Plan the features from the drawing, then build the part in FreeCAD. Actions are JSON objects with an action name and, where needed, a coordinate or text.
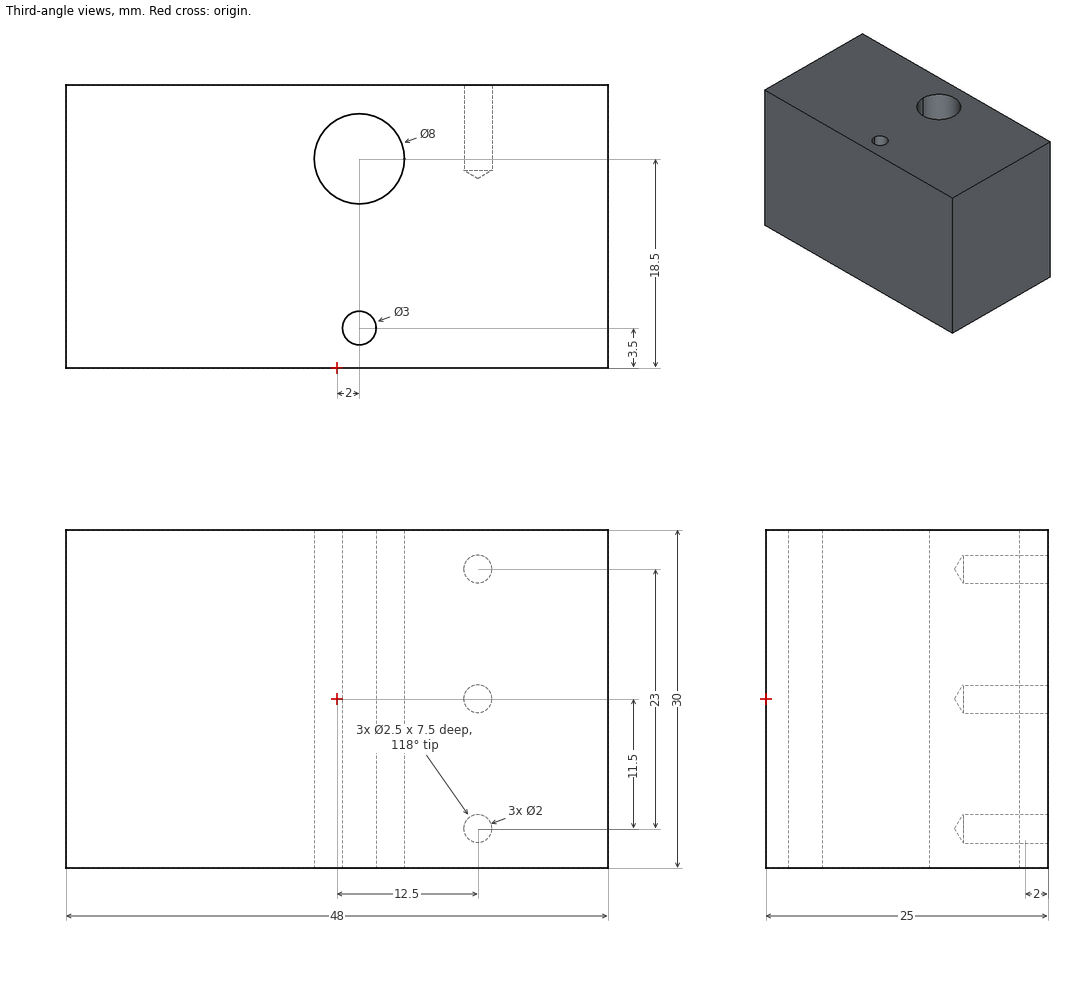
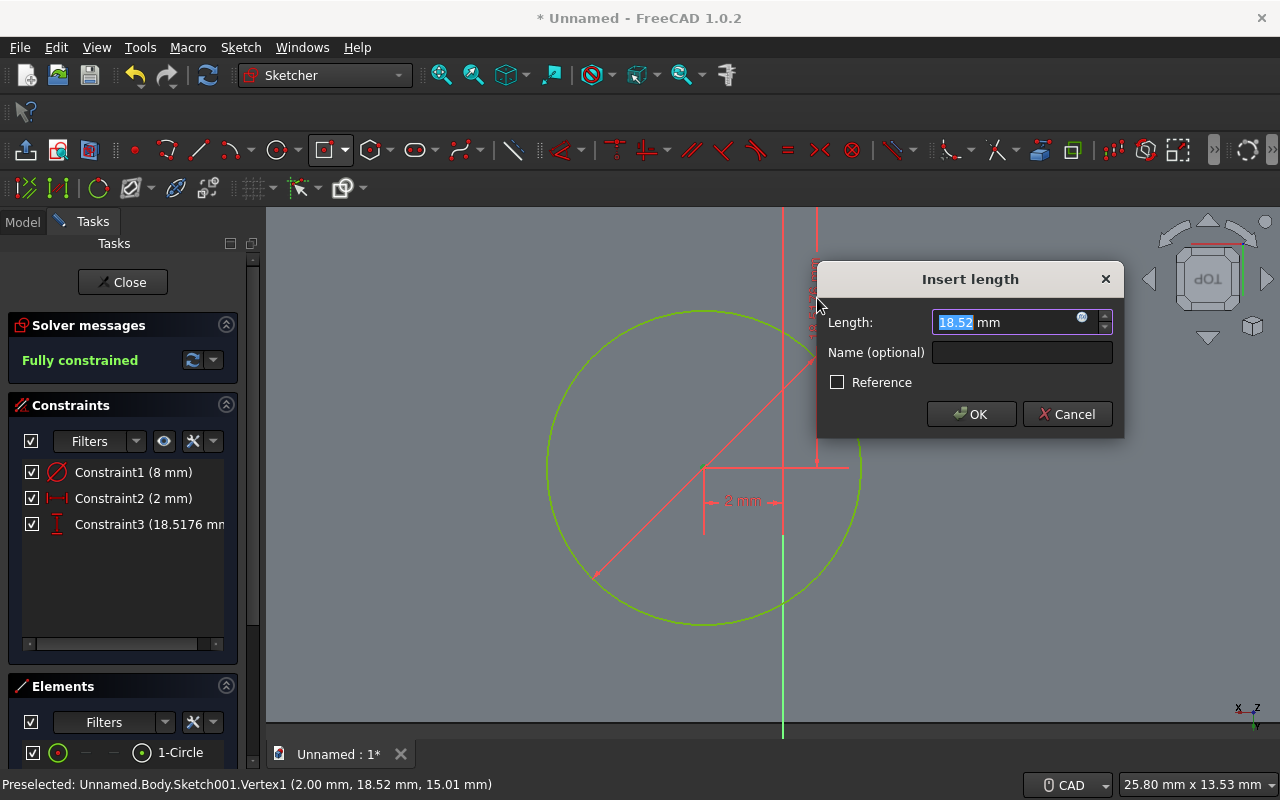
{"action": "type", "text": "18.5"}
{"action": "key", "text": "Return"}
{"action": "key", "text": "Escape"}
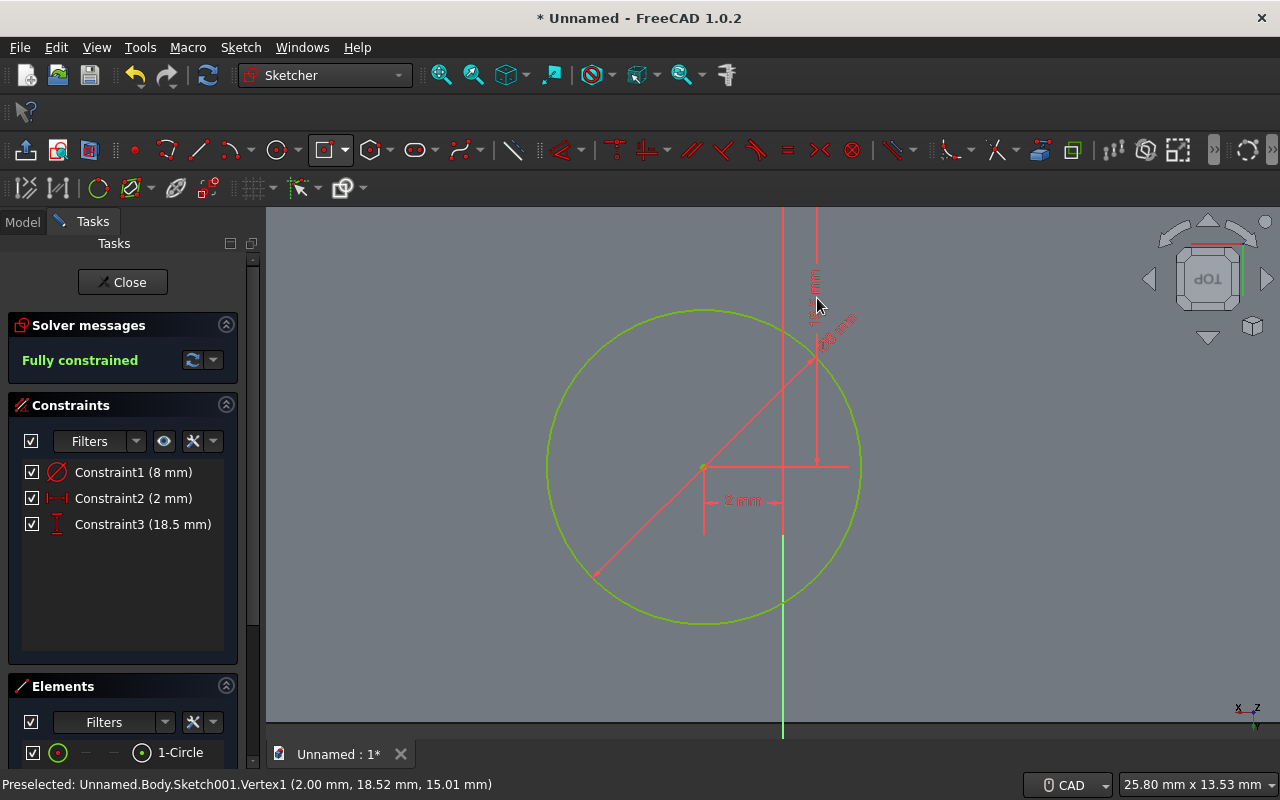
{"action": "left_click", "coordinate": [123, 282]}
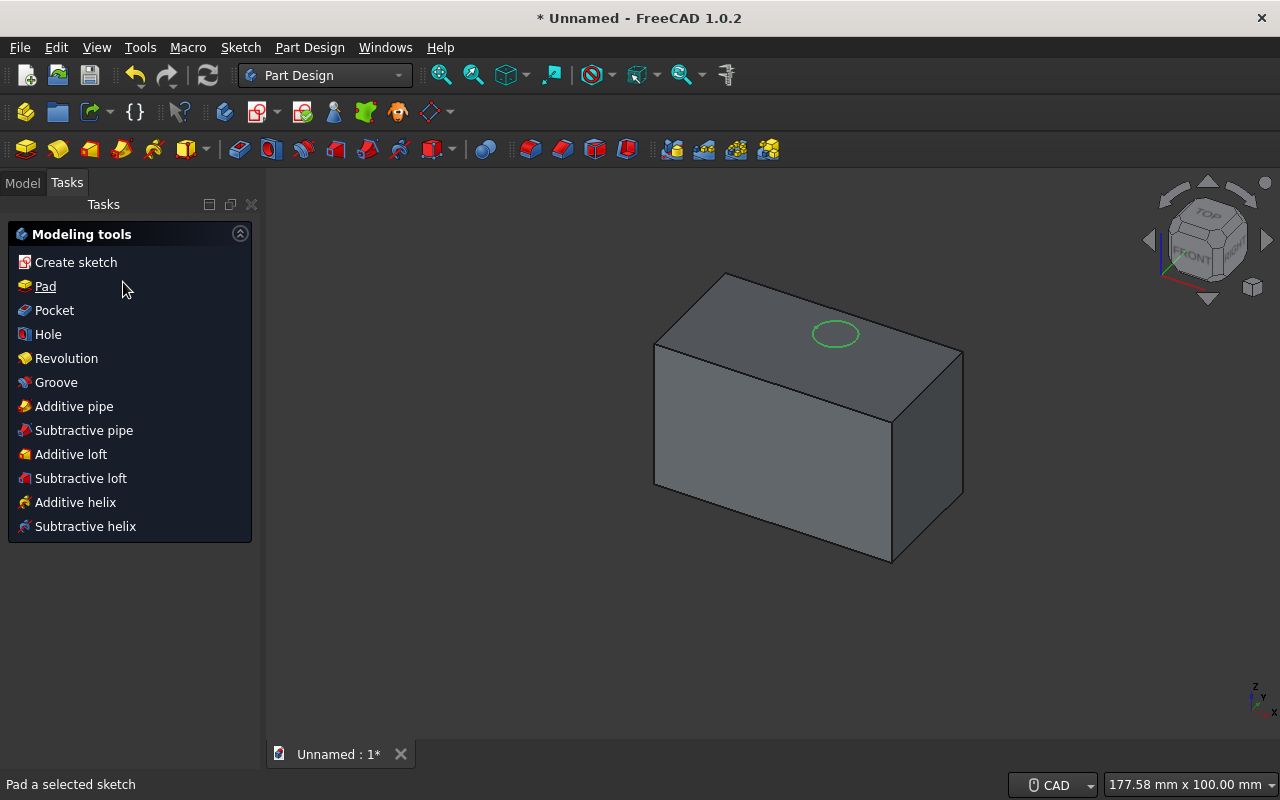
{"action": "left_click", "coordinate": [240, 150]}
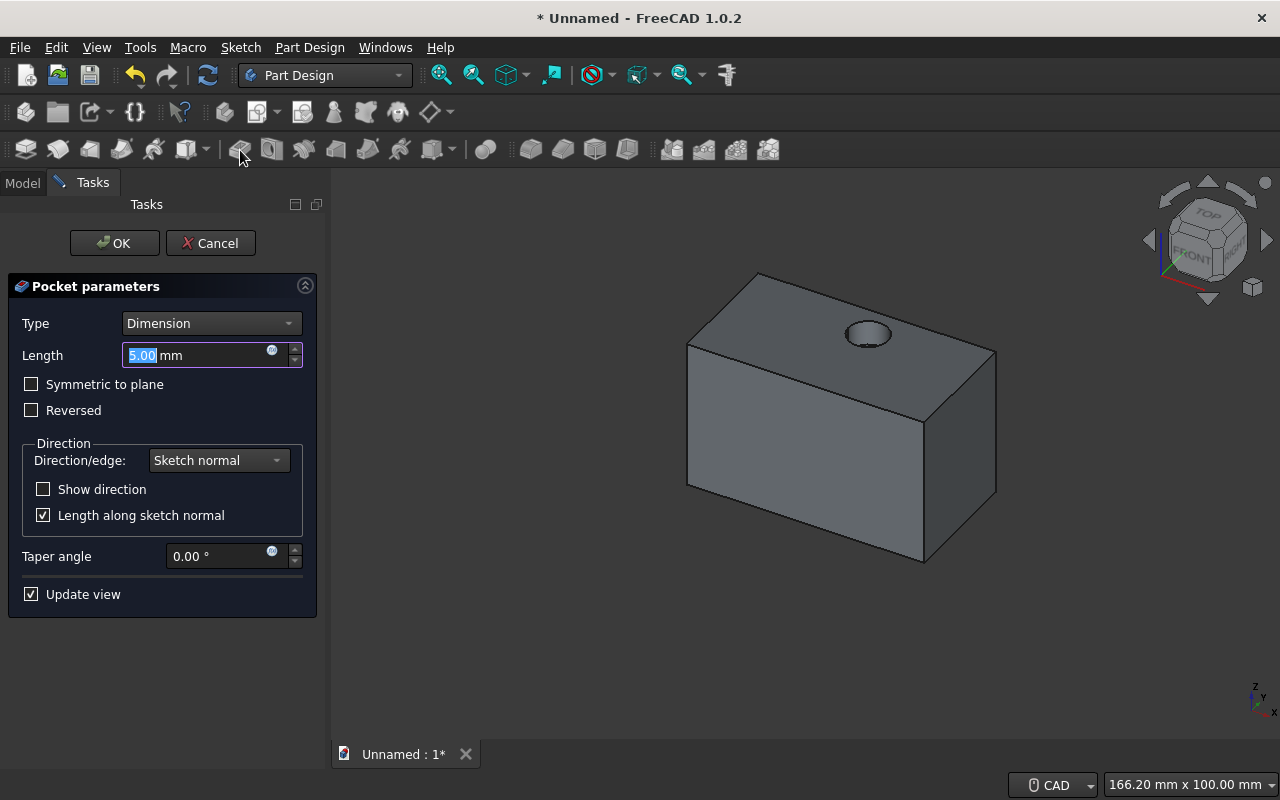
{"action": "left_click", "coordinate": [212, 324]}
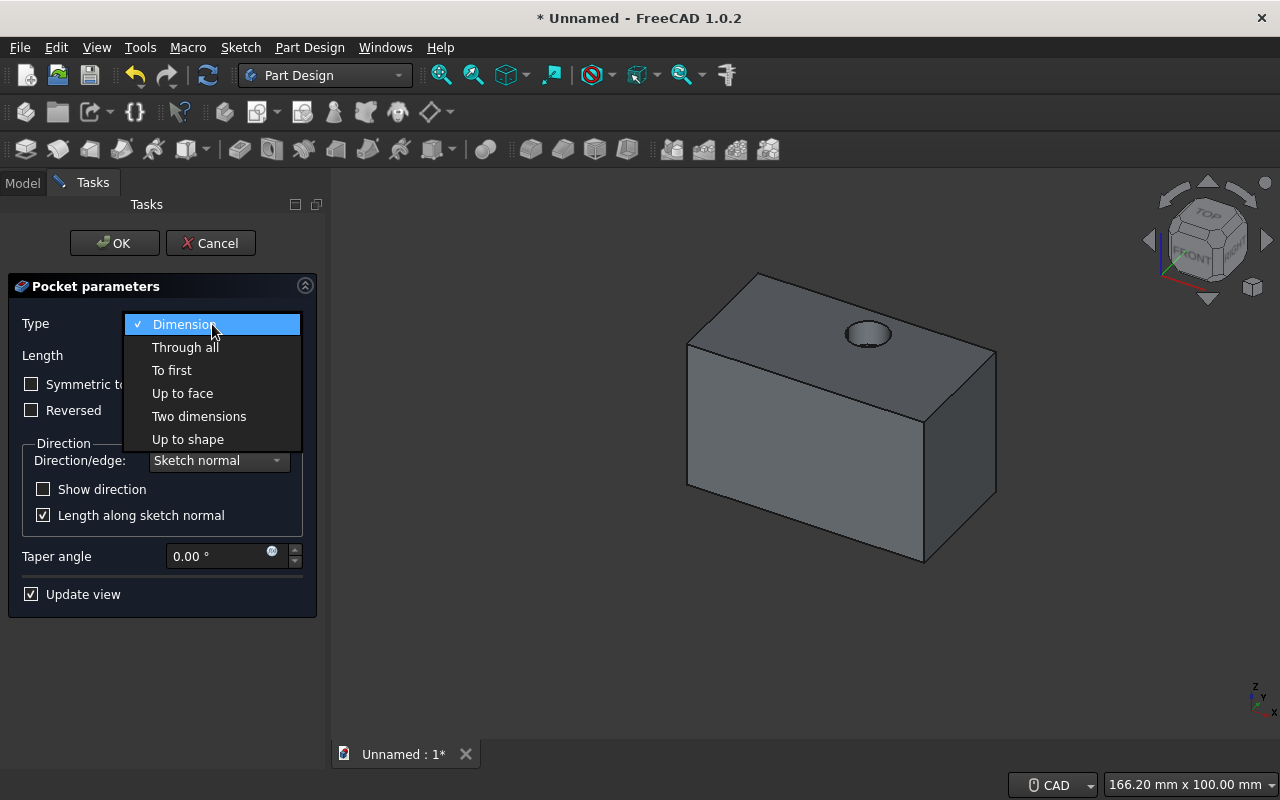
{"action": "left_click", "coordinate": [212, 370]}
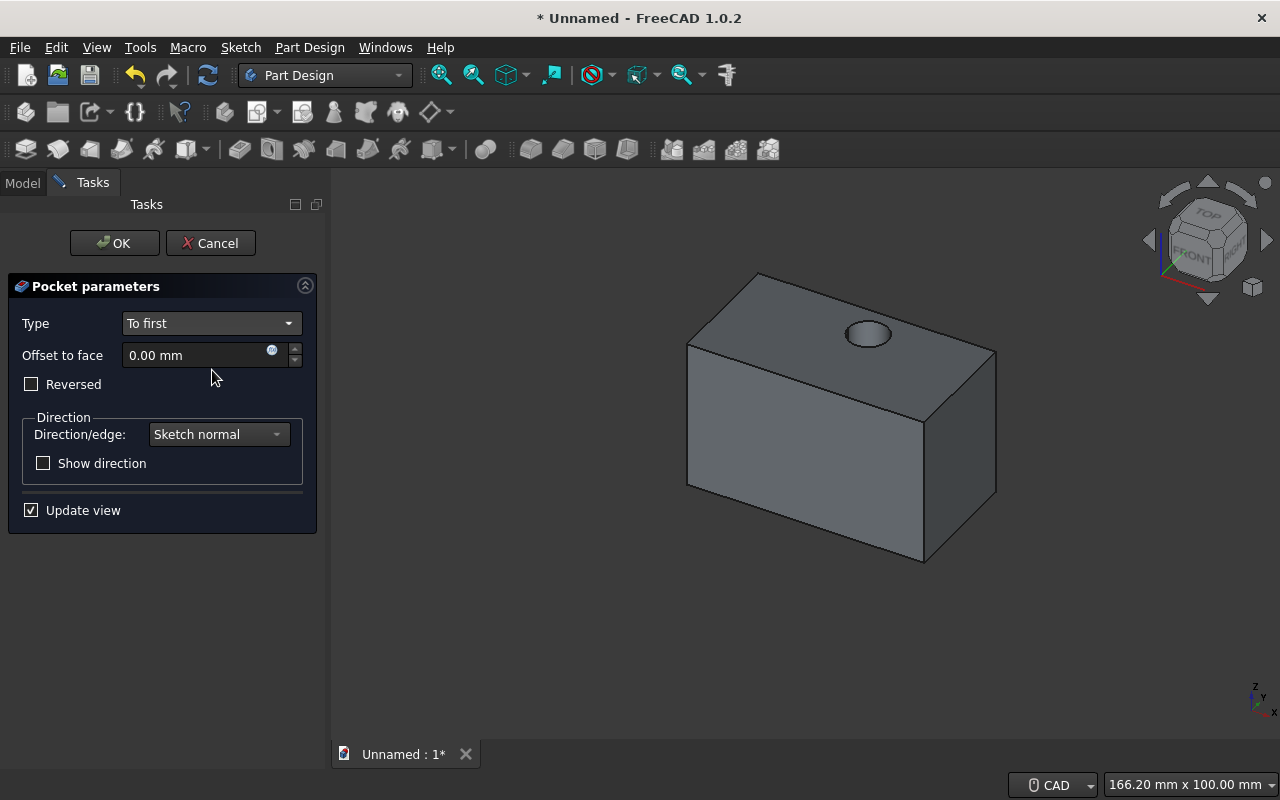
{"action": "left_click", "coordinate": [115, 243]}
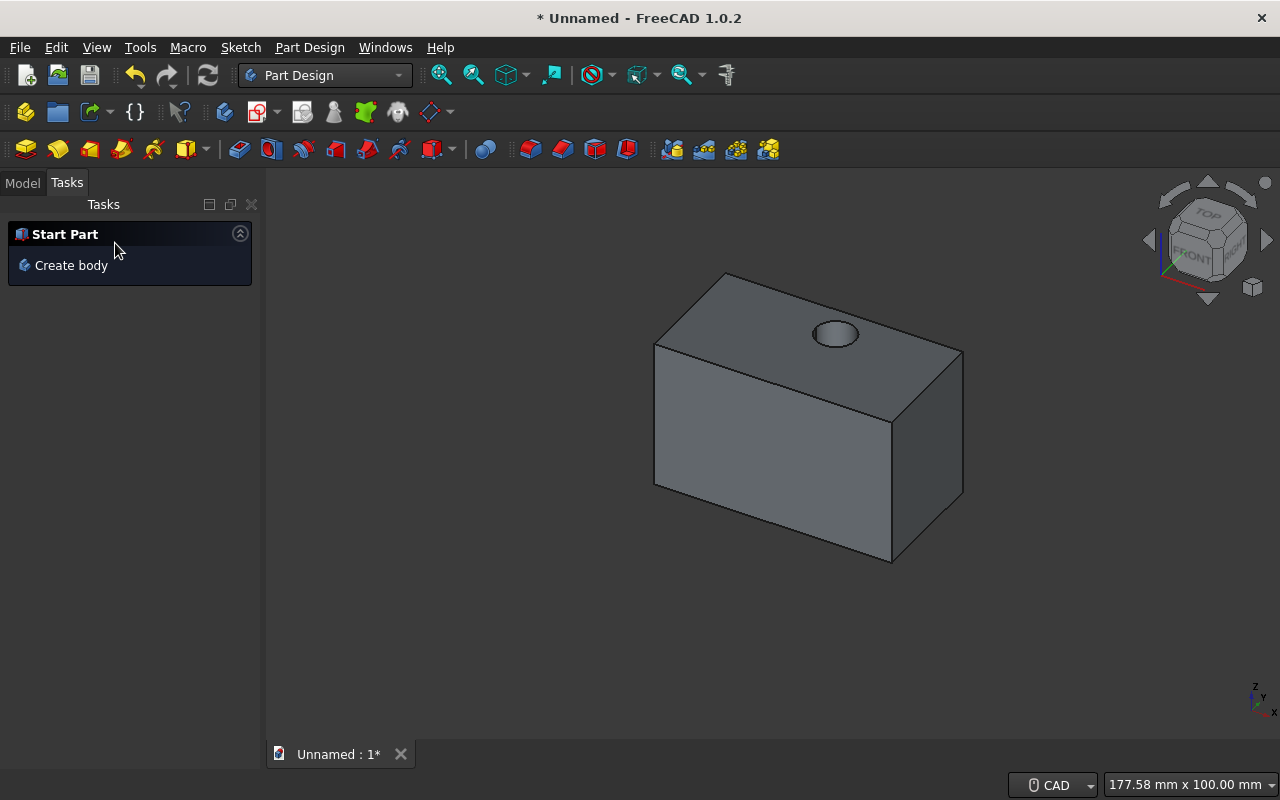
{"action": "left_click", "coordinate": [741, 324]}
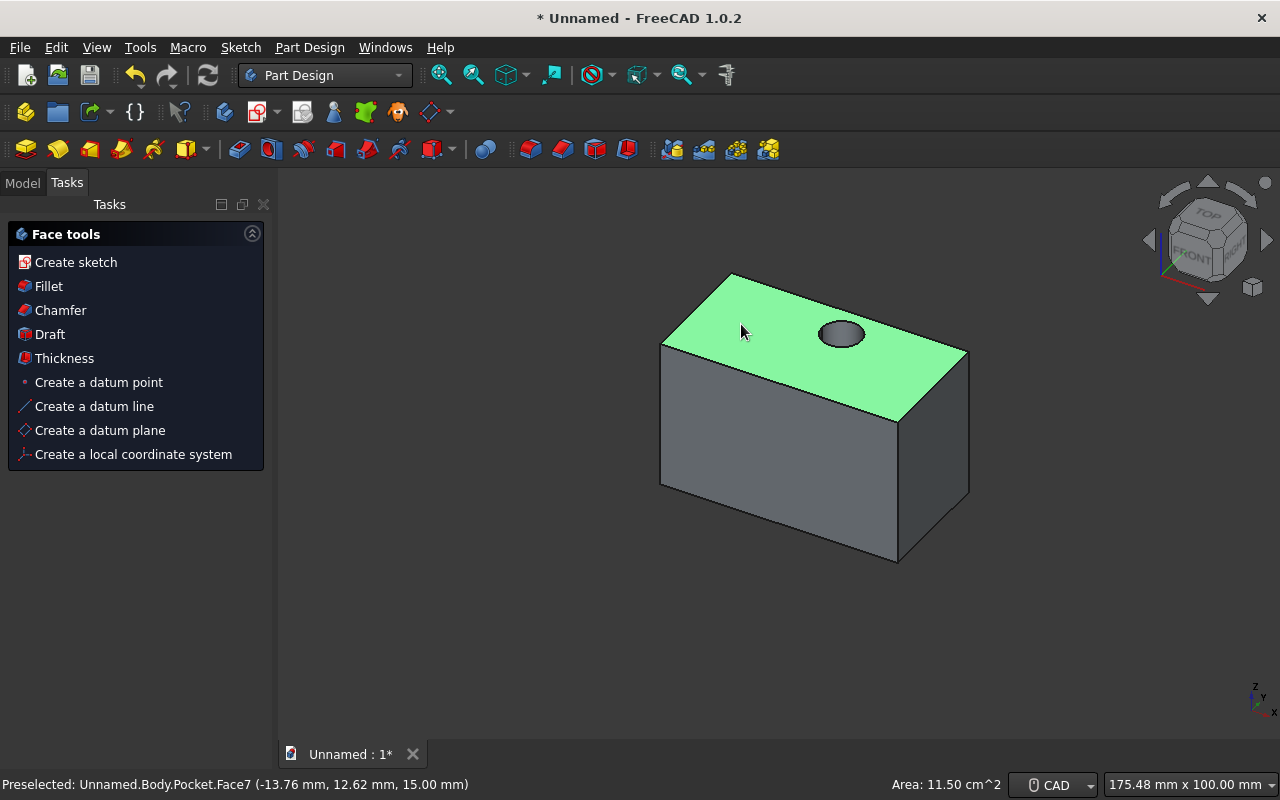
{"action": "left_click", "coordinate": [258, 112]}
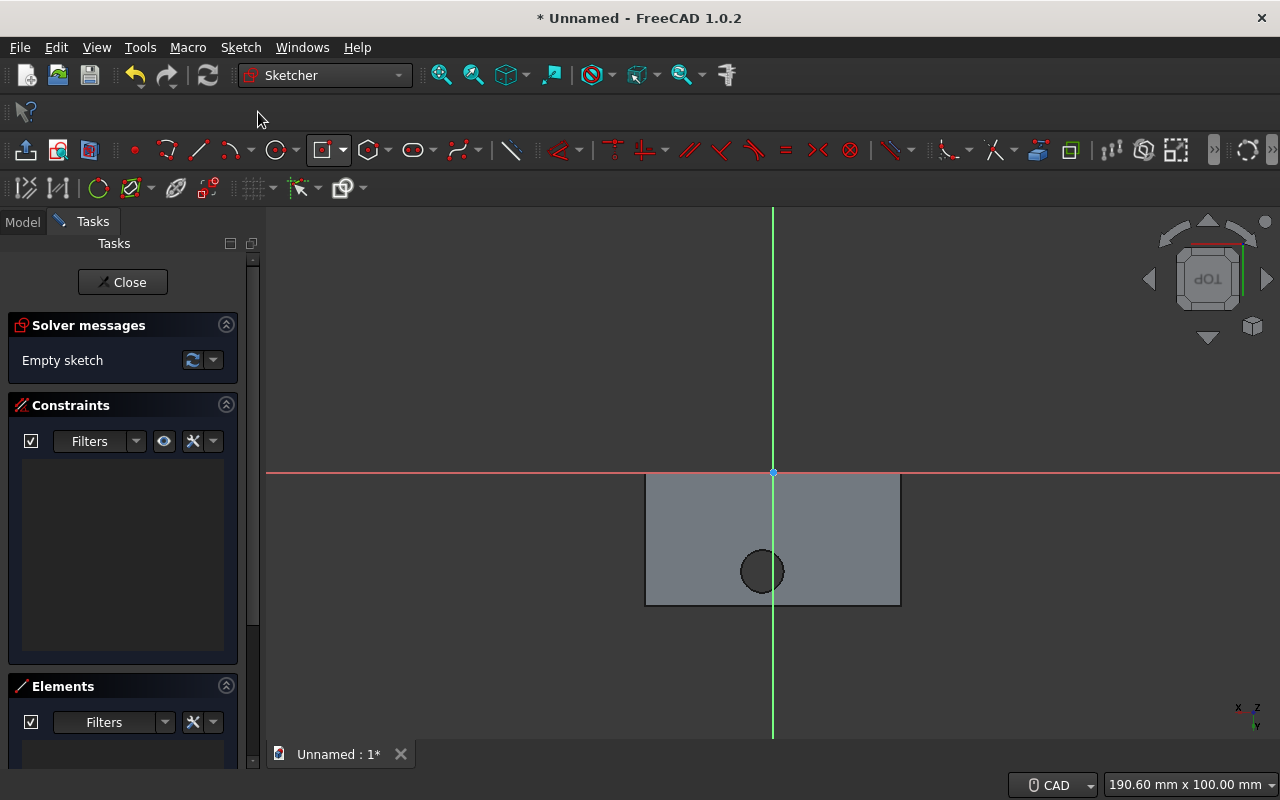
{"action": "scroll", "coordinate": [768, 487], "scroll_direction": "up", "scroll_amount": 13}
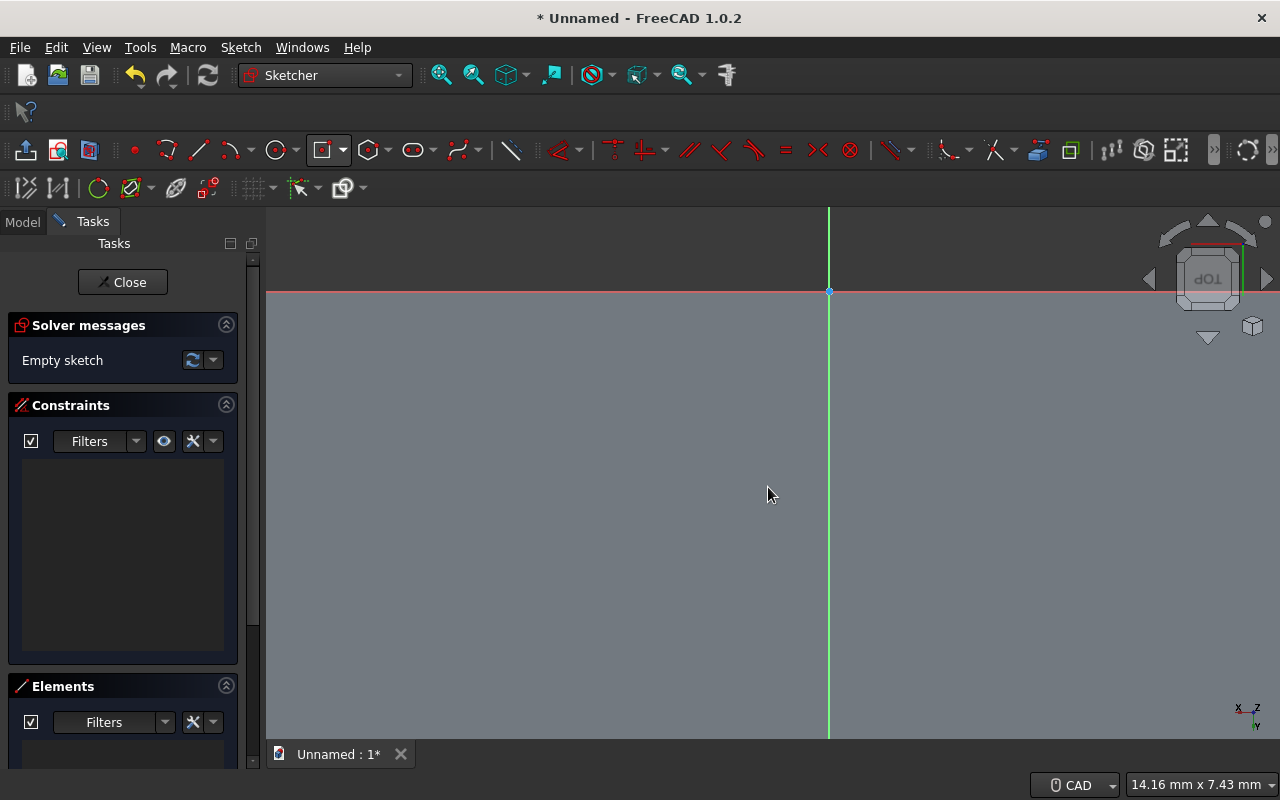
{"action": "key", "text": "g c"}